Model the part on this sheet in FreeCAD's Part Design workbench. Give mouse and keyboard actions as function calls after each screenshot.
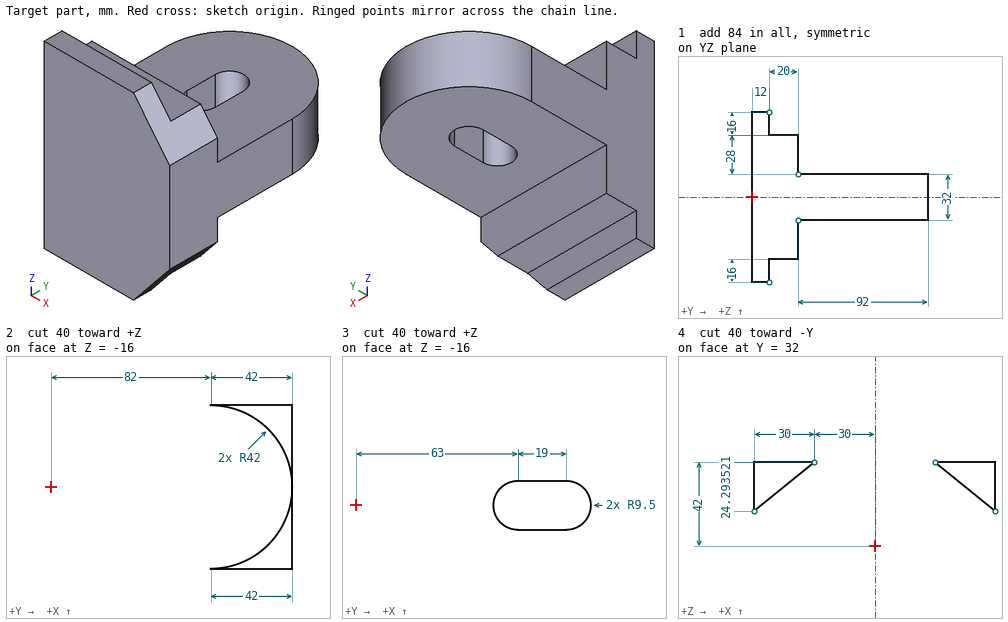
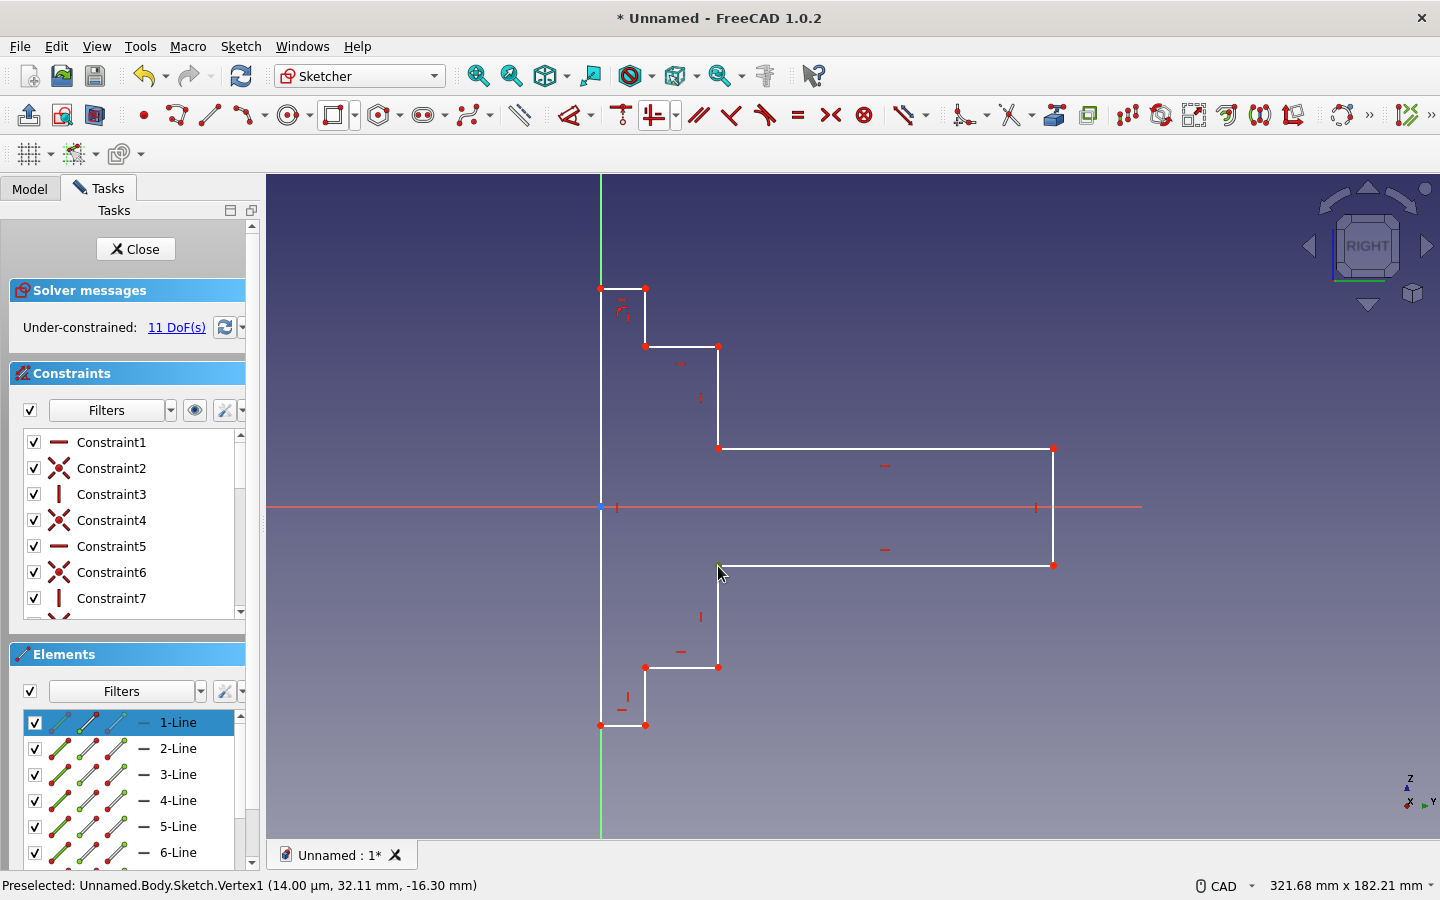
click(718, 449)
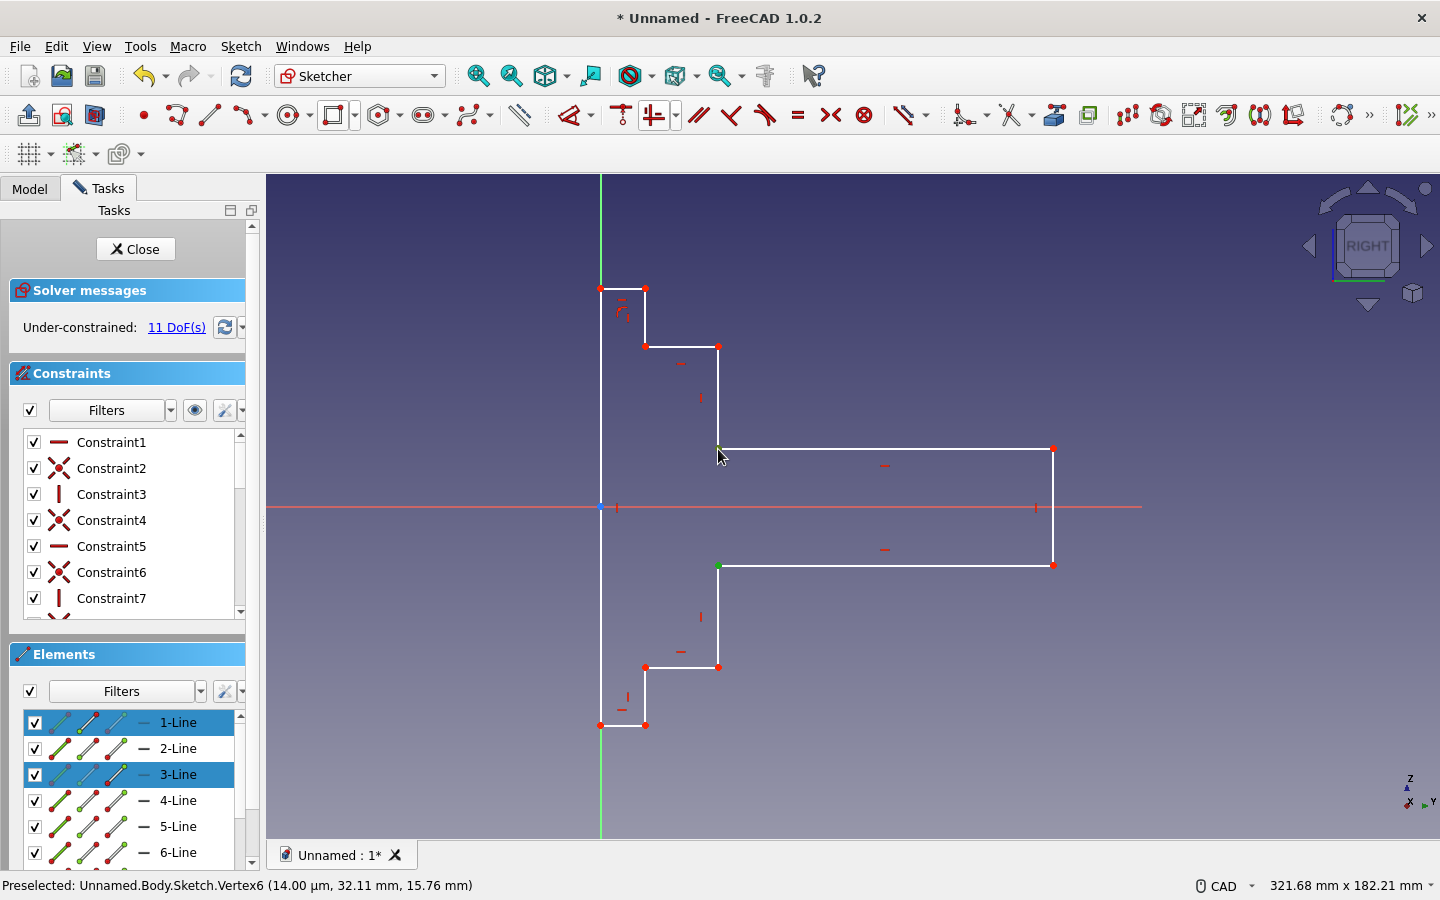
click(364, 506)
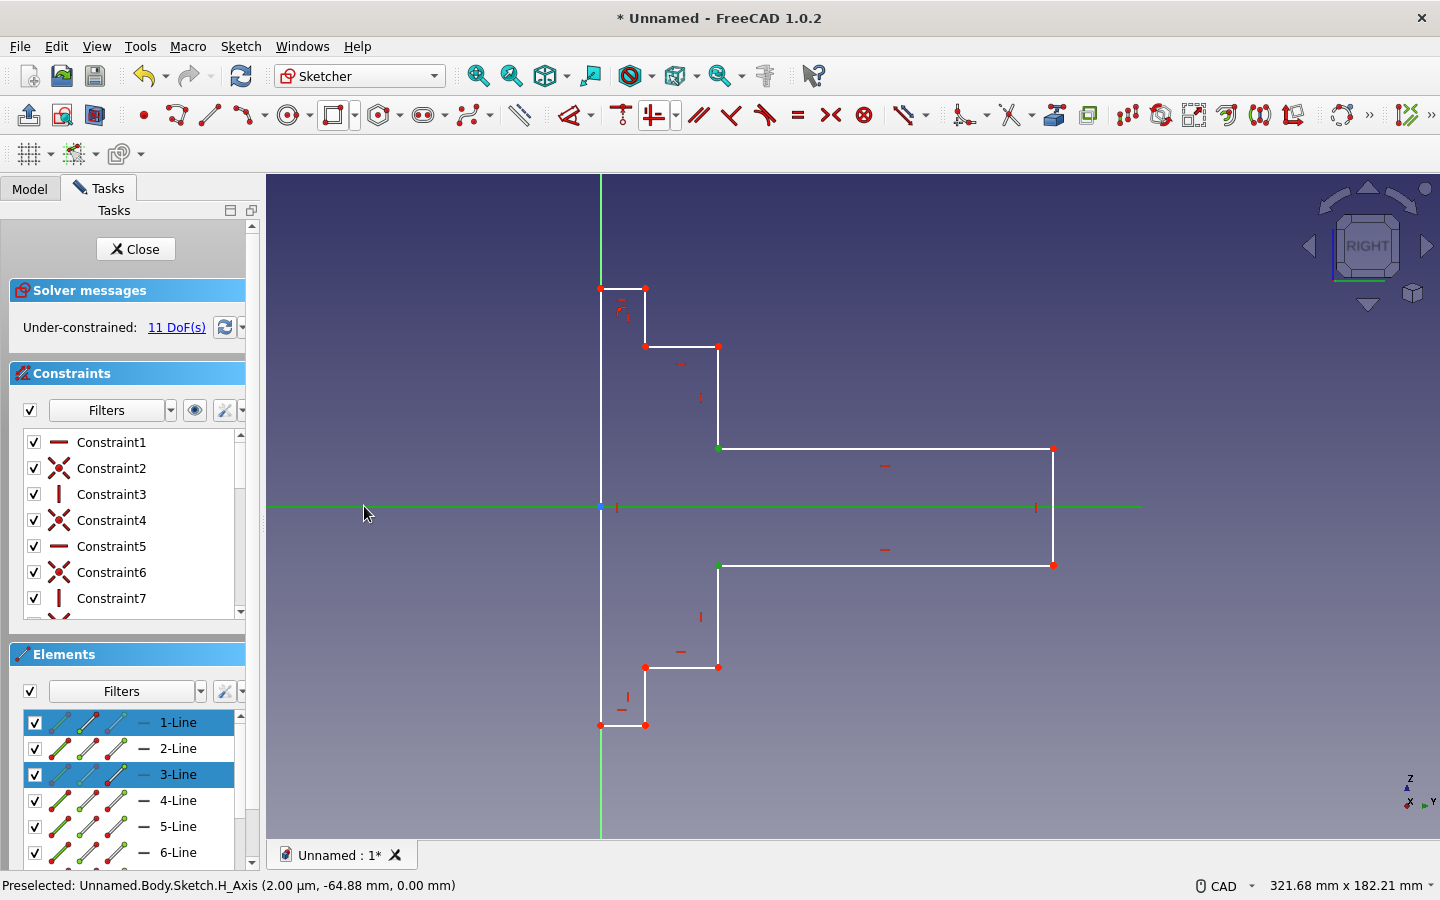
key(s)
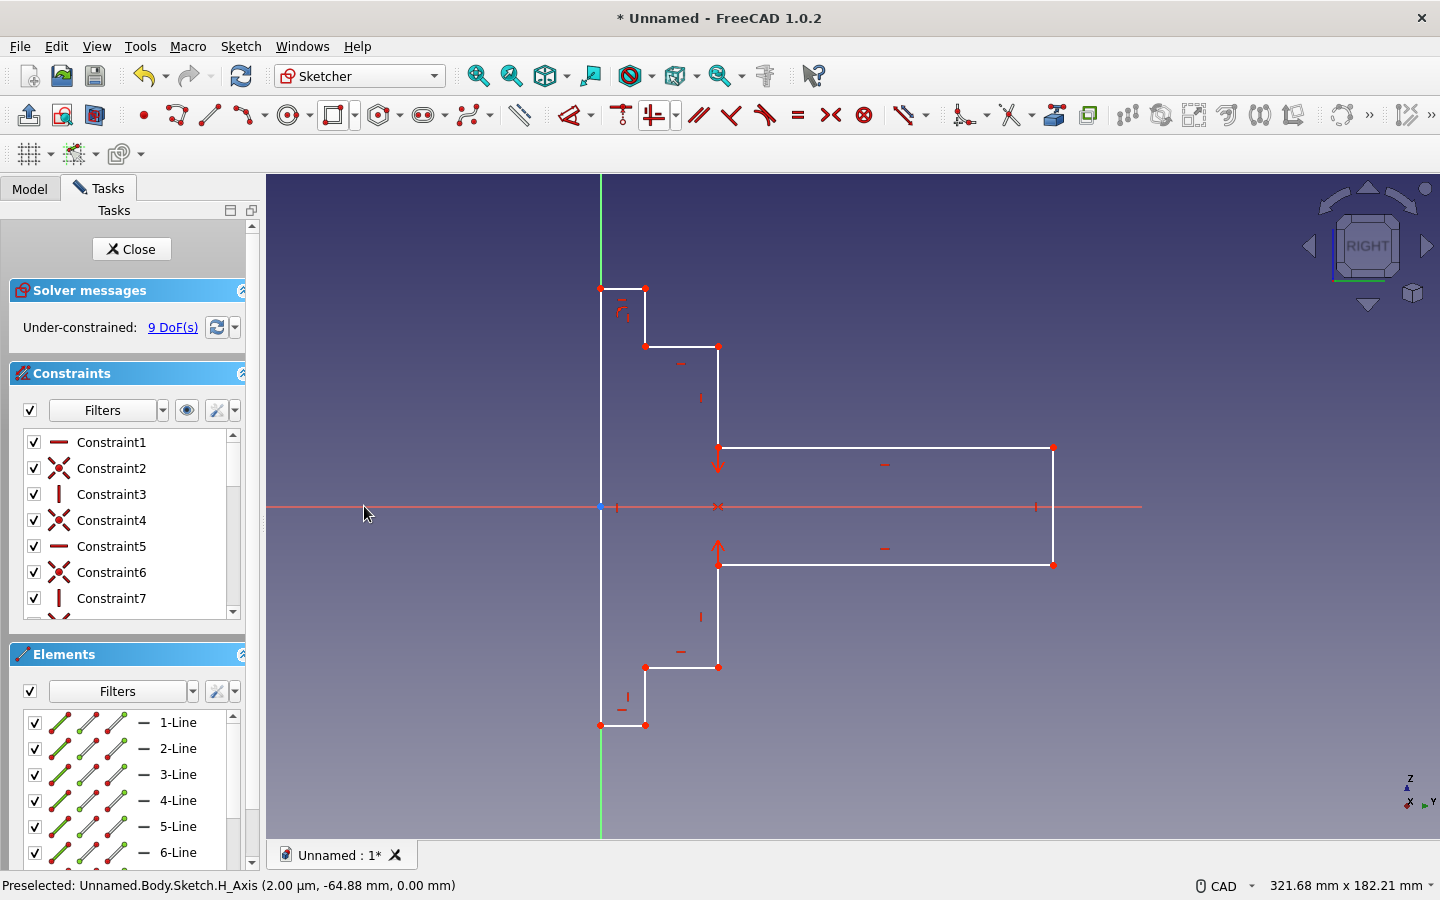
click(645, 289)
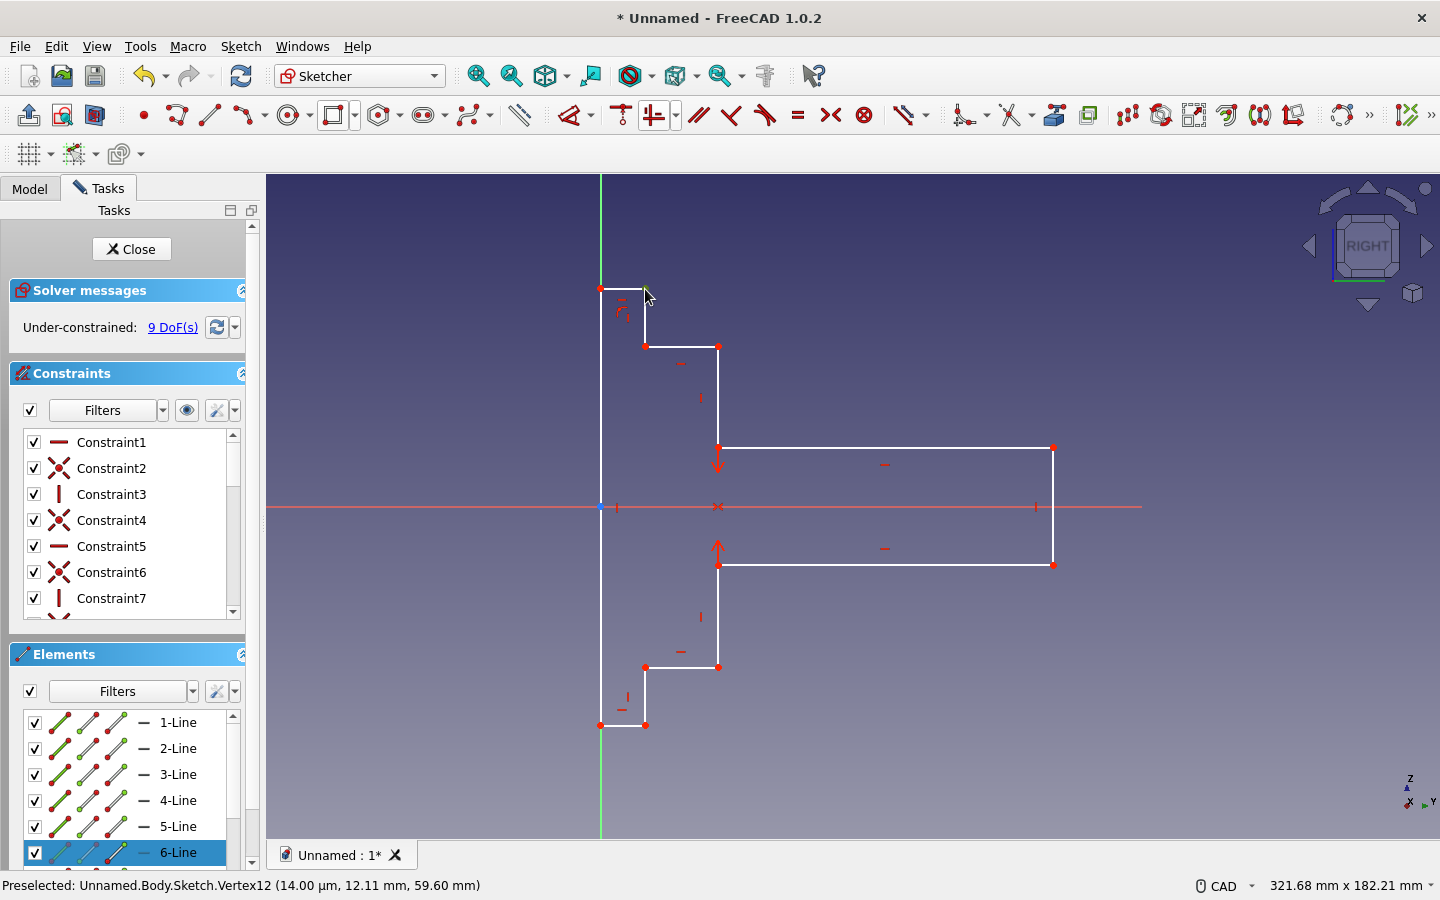
click(645, 726)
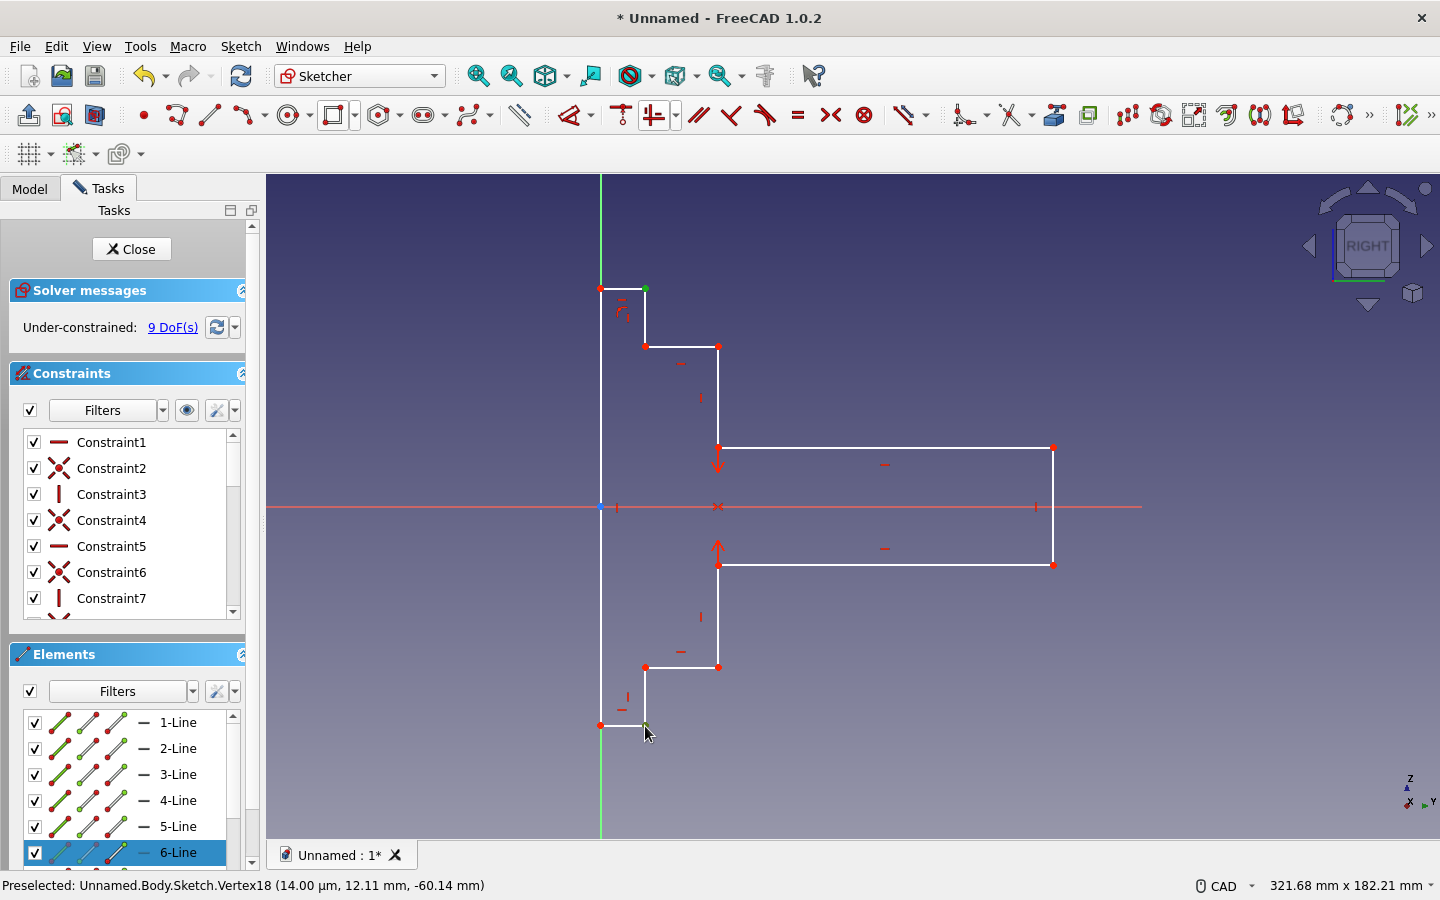
click(364, 506)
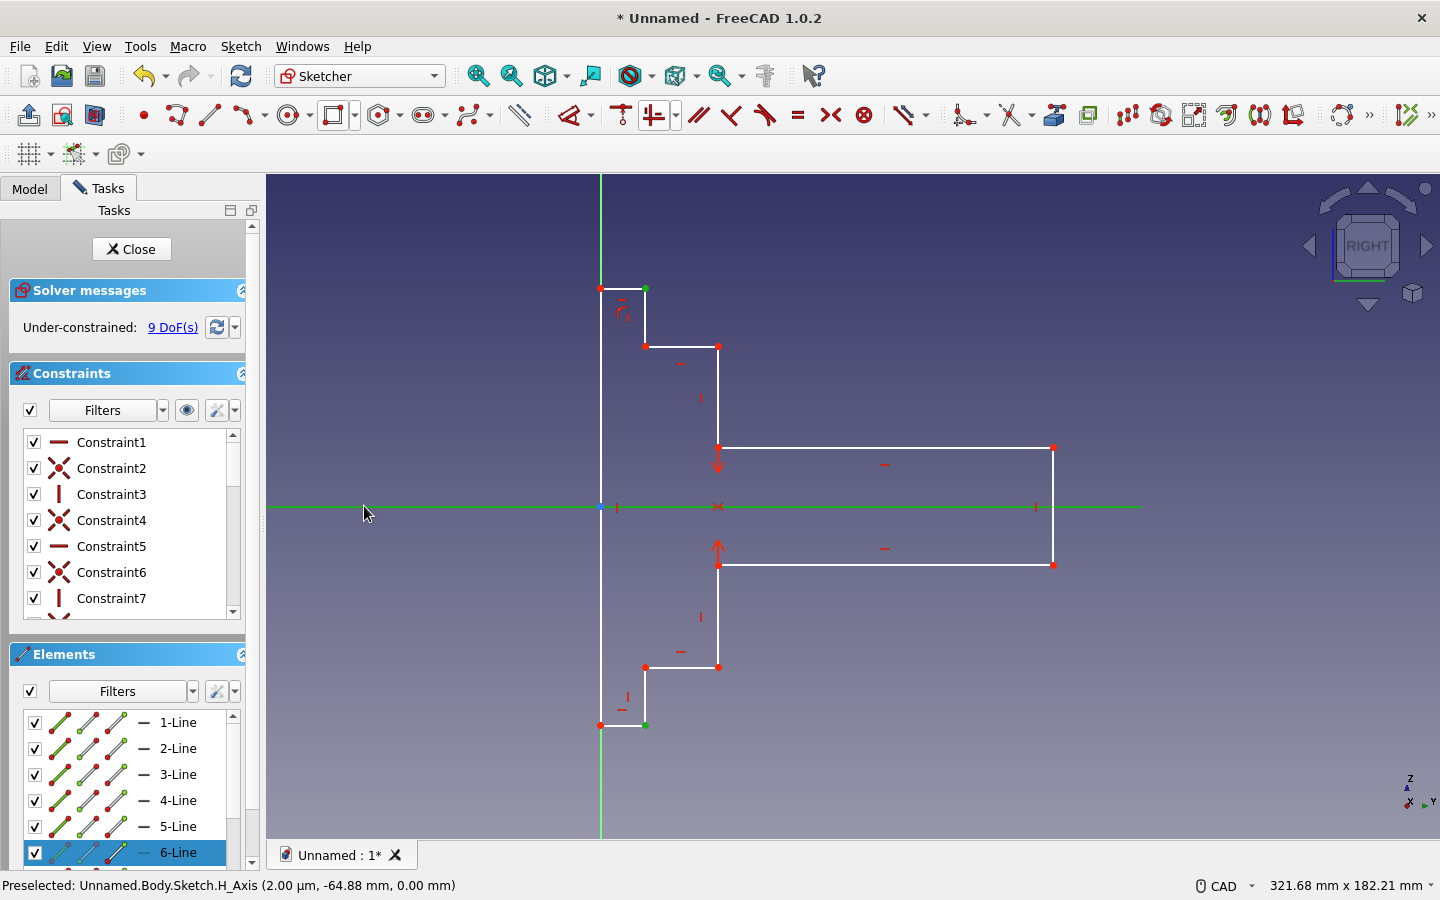
key(s)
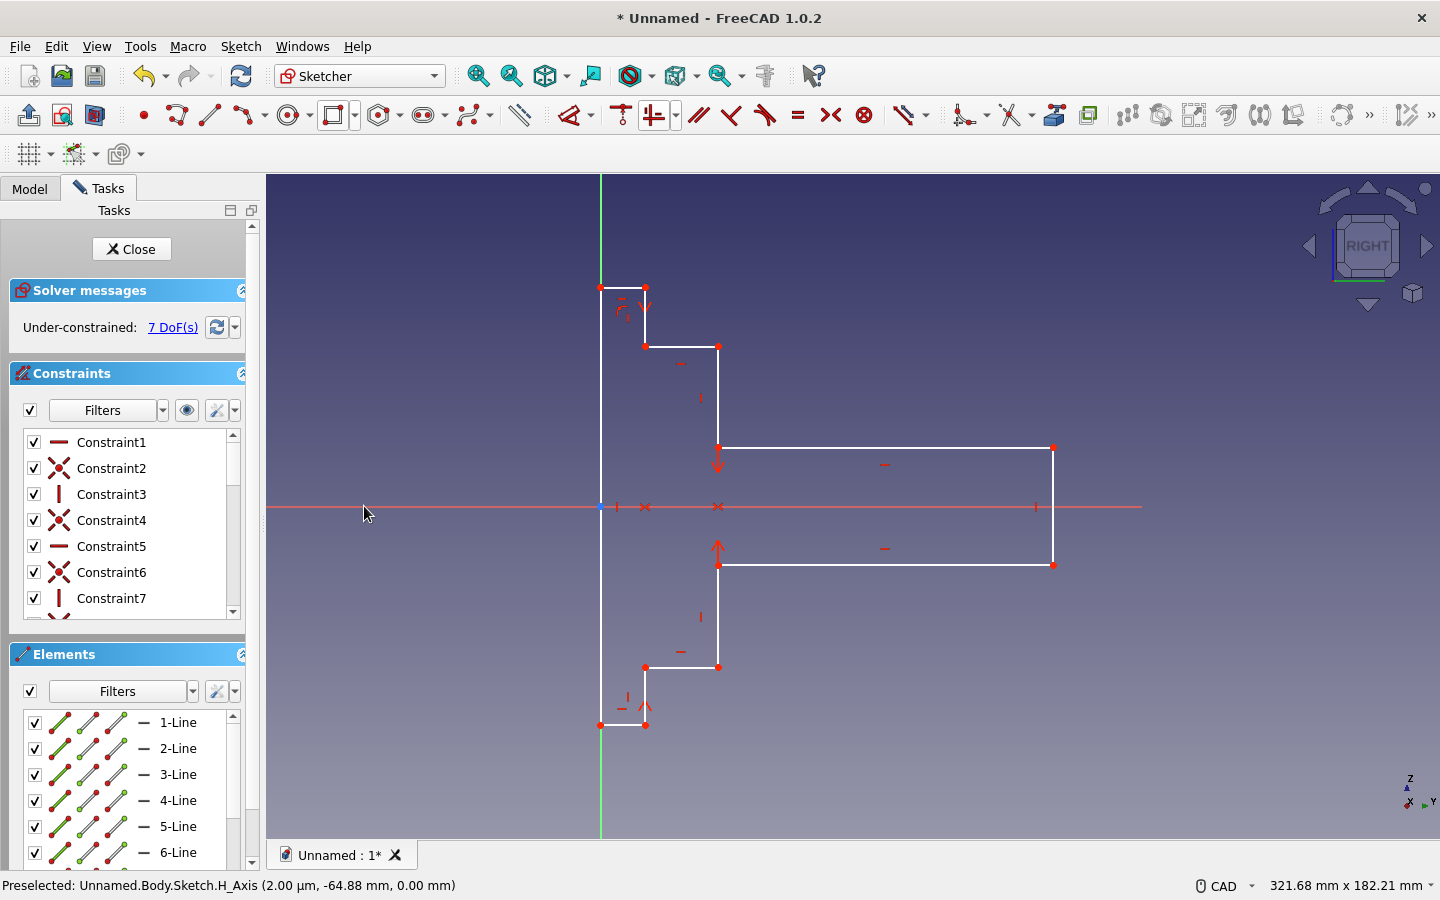
click(819, 565)